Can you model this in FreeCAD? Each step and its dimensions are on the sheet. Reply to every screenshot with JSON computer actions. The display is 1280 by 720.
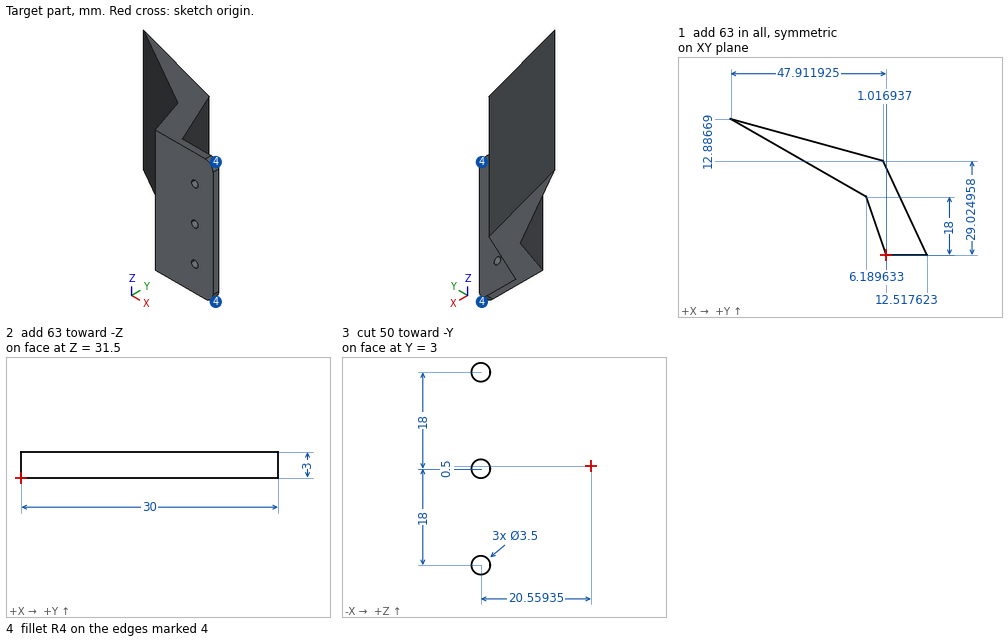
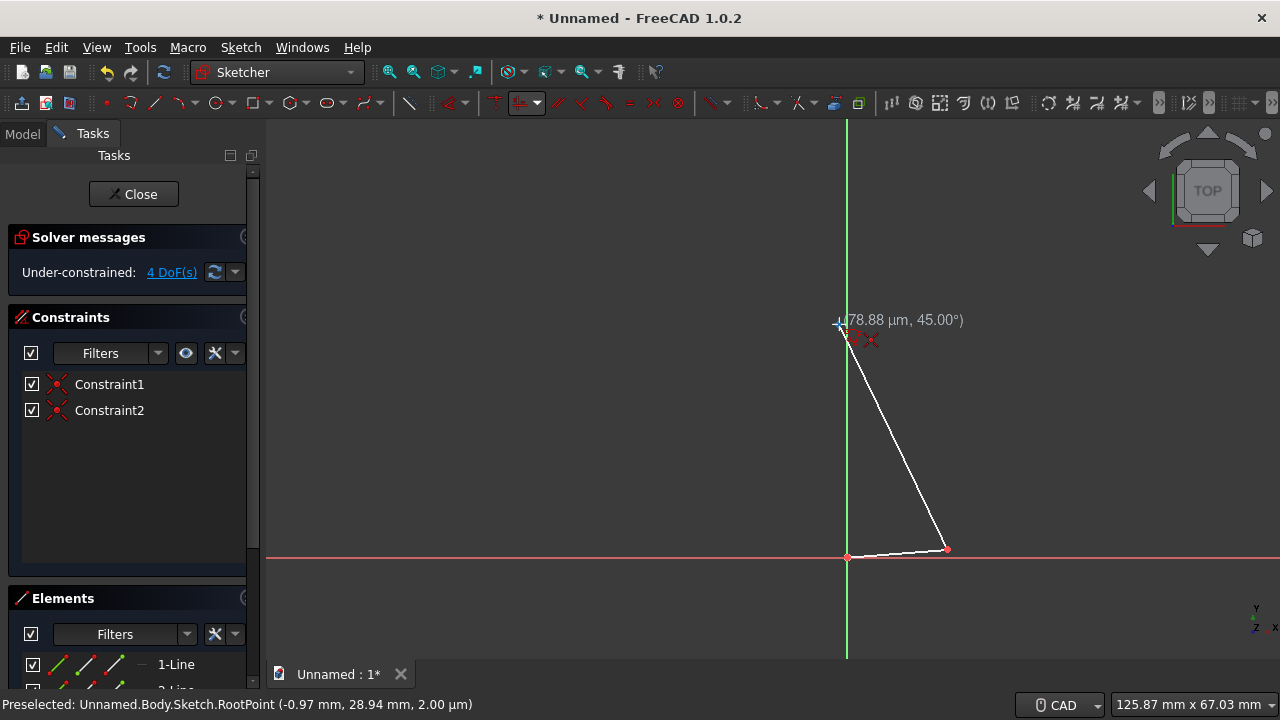
{"action": "left_click", "coordinate": [461, 220]}
{"action": "left_click", "coordinate": [797, 413]}
{"action": "left_click", "coordinate": [847, 558]}
{"action": "key", "text": "Escape"}
{"action": "key", "text": "Escape"}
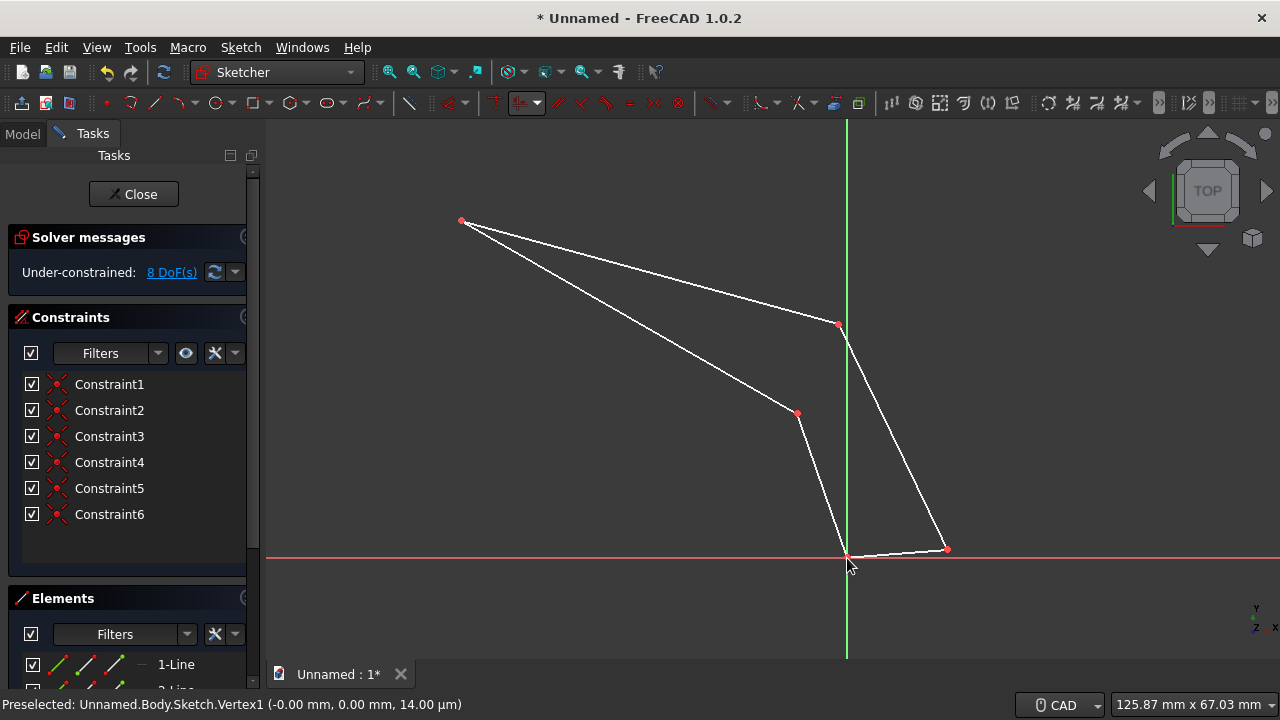
{"action": "left_click", "coordinate": [877, 555]}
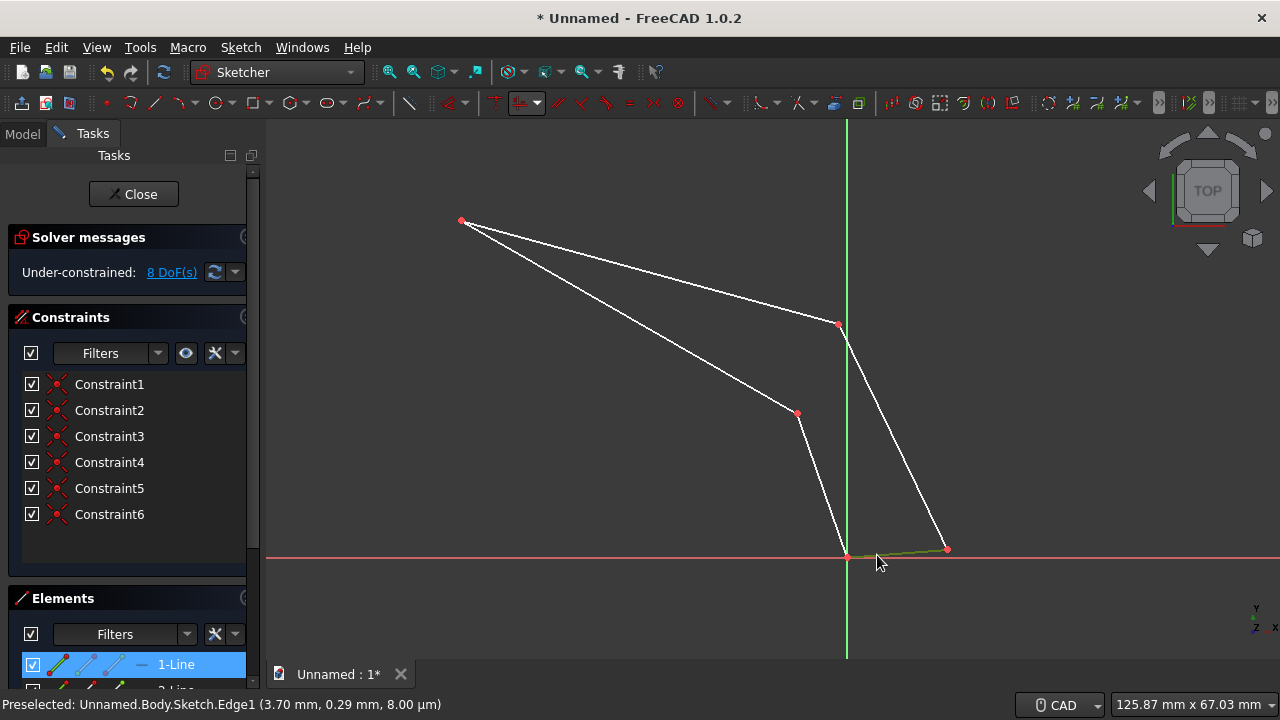
{"action": "key", "text": "h"}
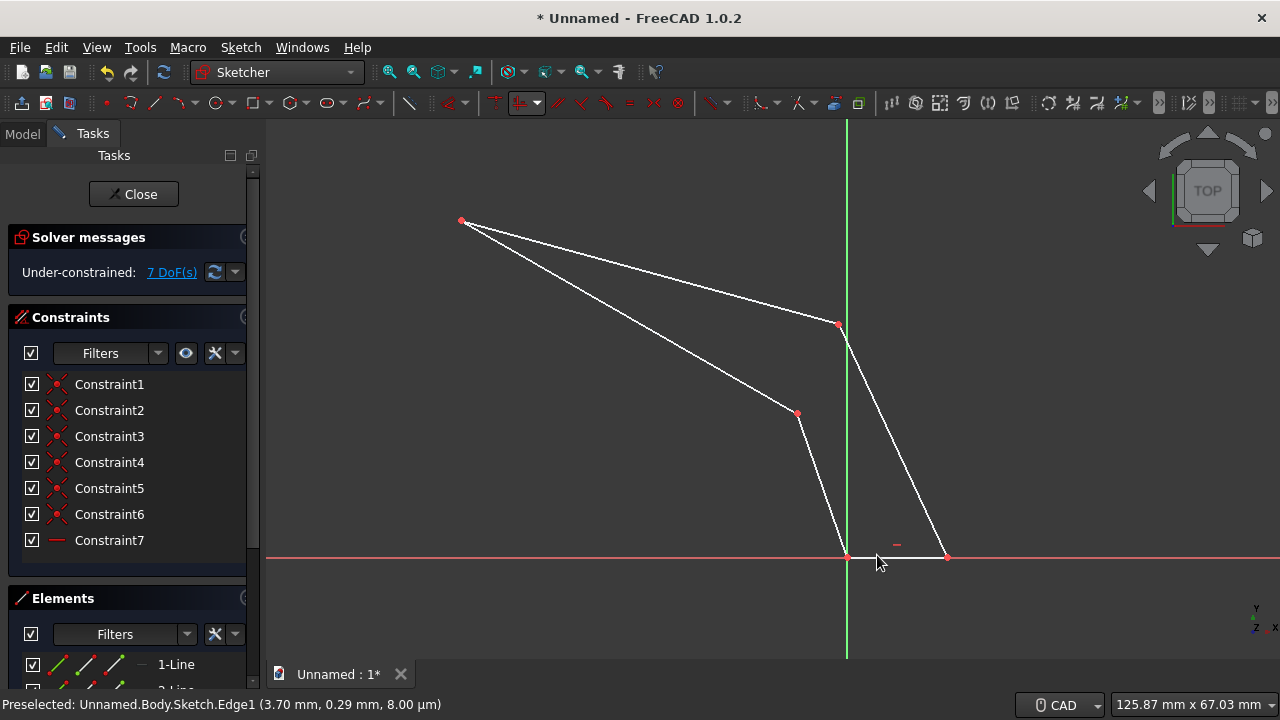
{"action": "key", "text": "d"}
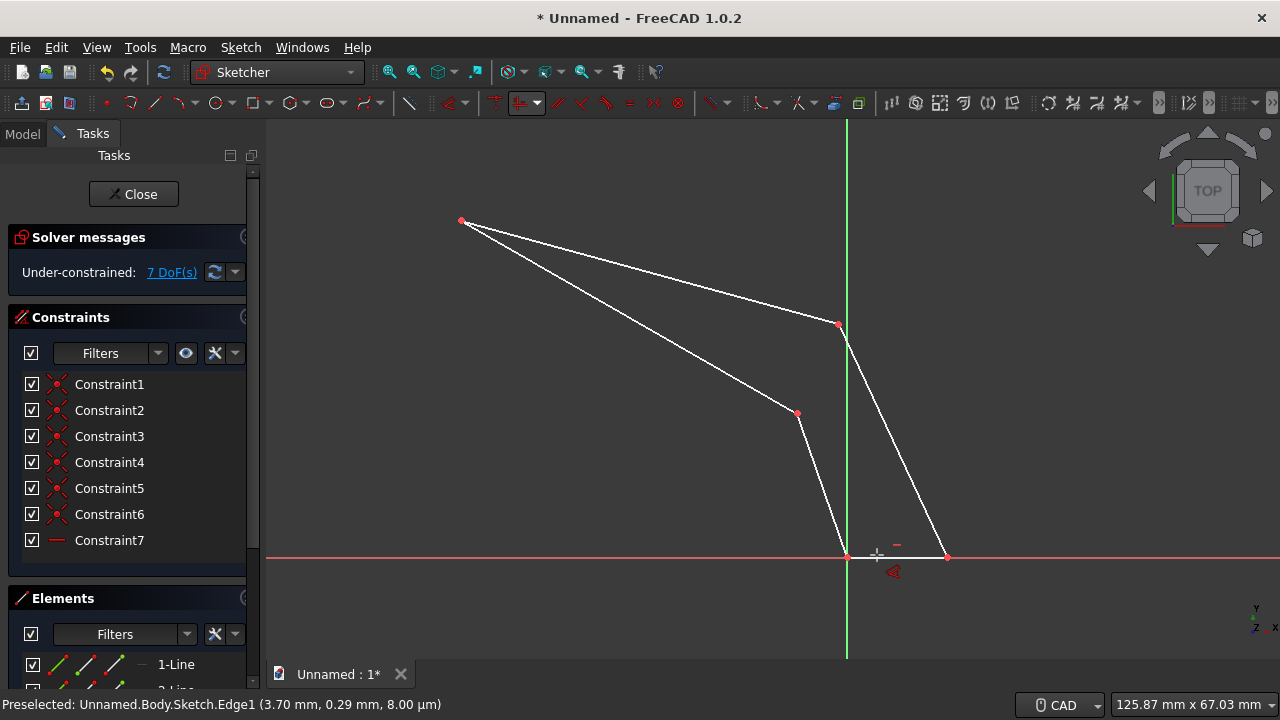
{"action": "left_click", "coordinate": [797, 414]}
{"action": "left_click", "coordinate": [881, 486]}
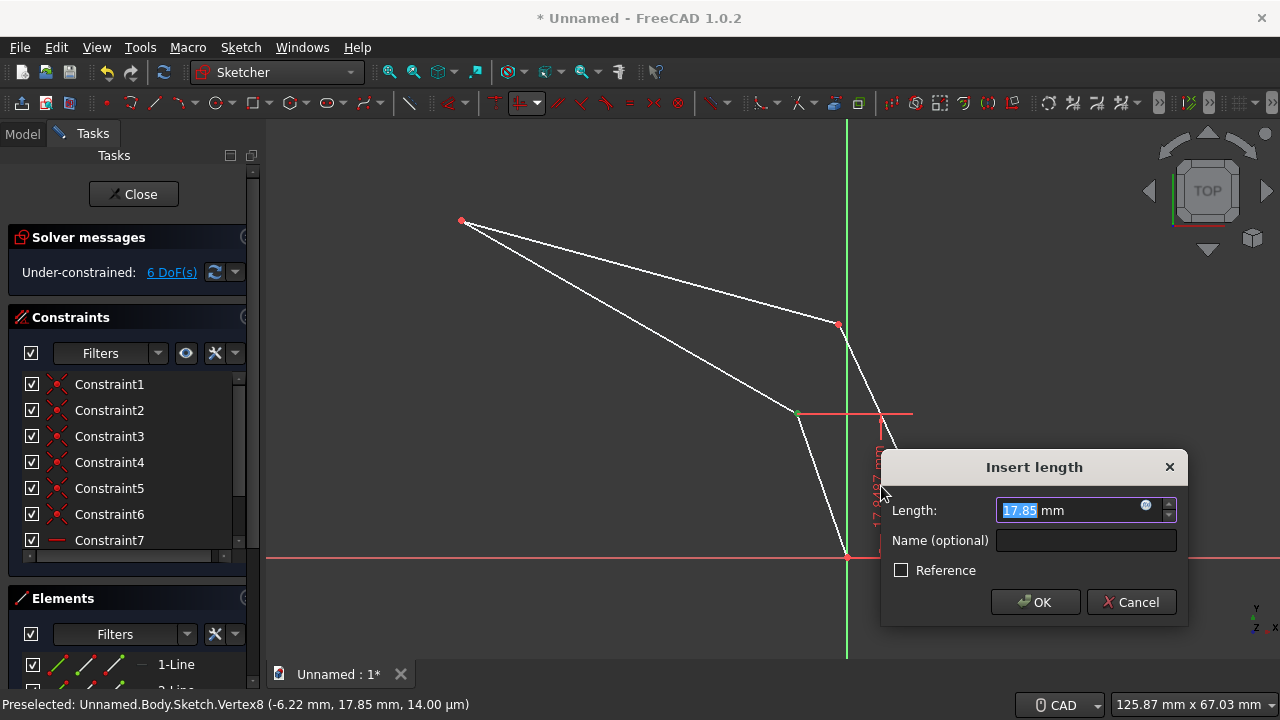
{"action": "type", "text": "18"}
{"action": "key", "text": "Return"}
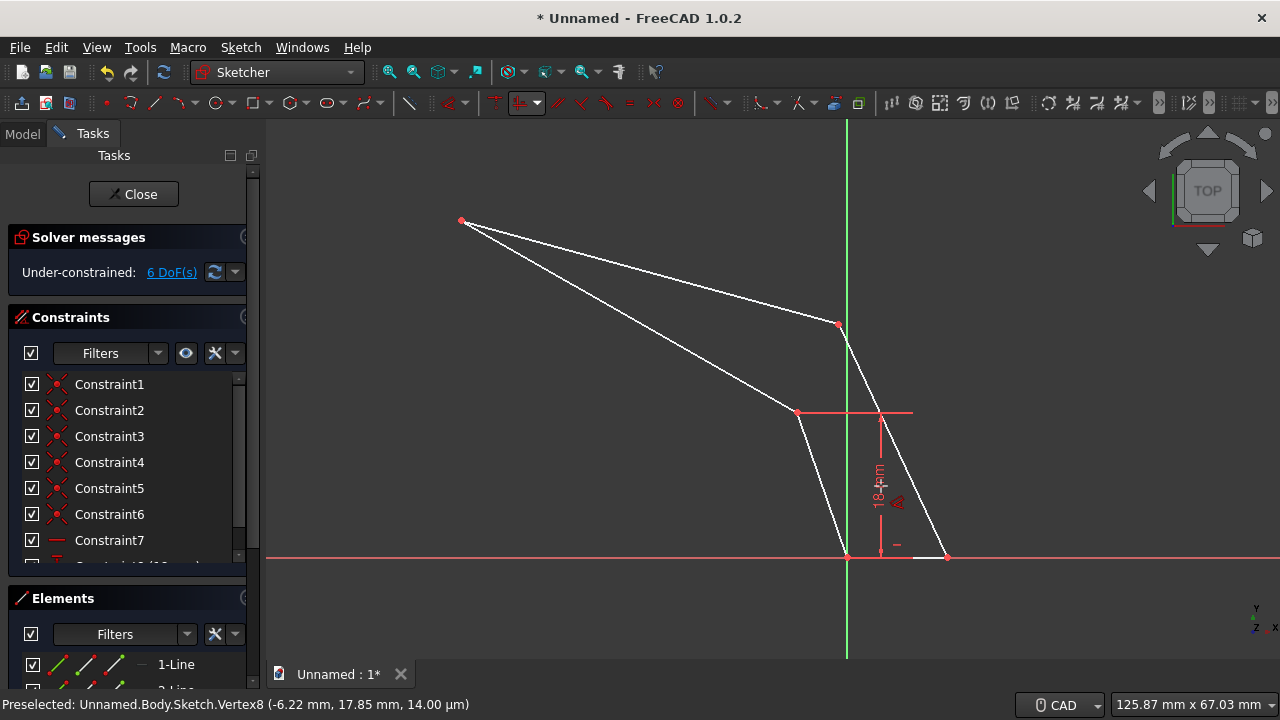
{"action": "left_click", "coordinate": [877, 558]}
{"action": "left_click", "coordinate": [897, 592]}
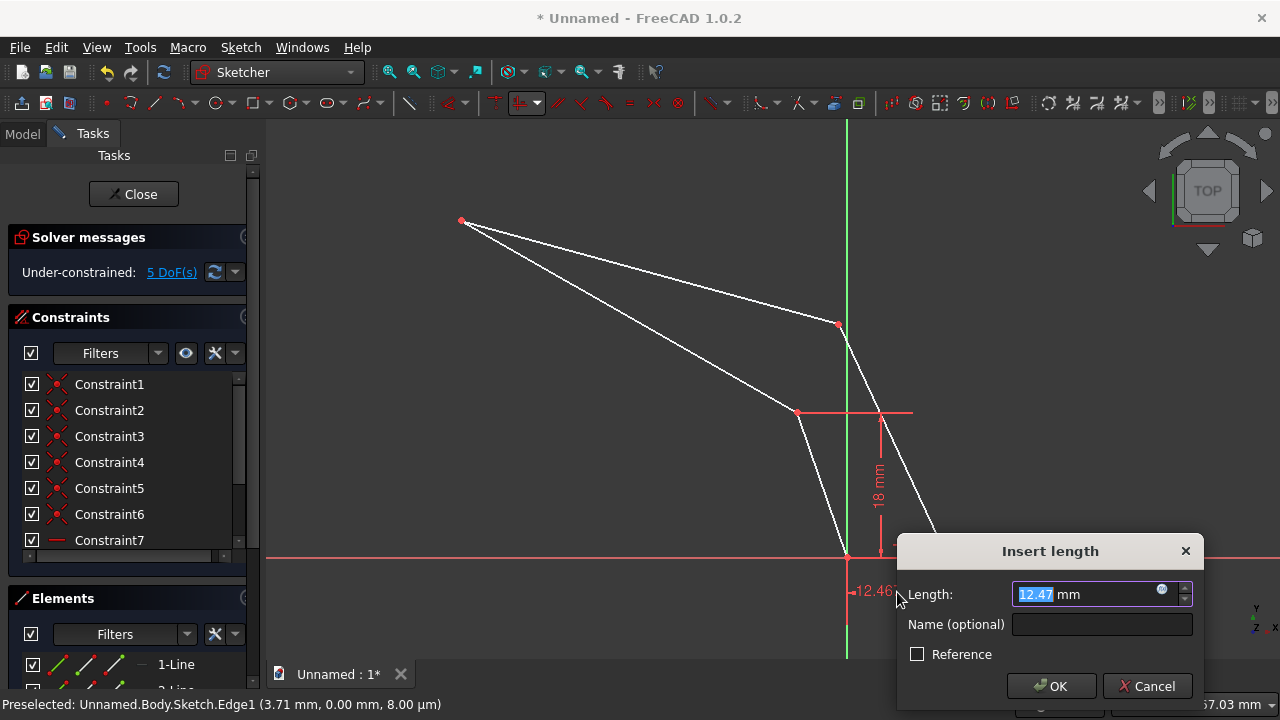
{"action": "type", "text": "12.517623"}
{"action": "key", "text": "Return"}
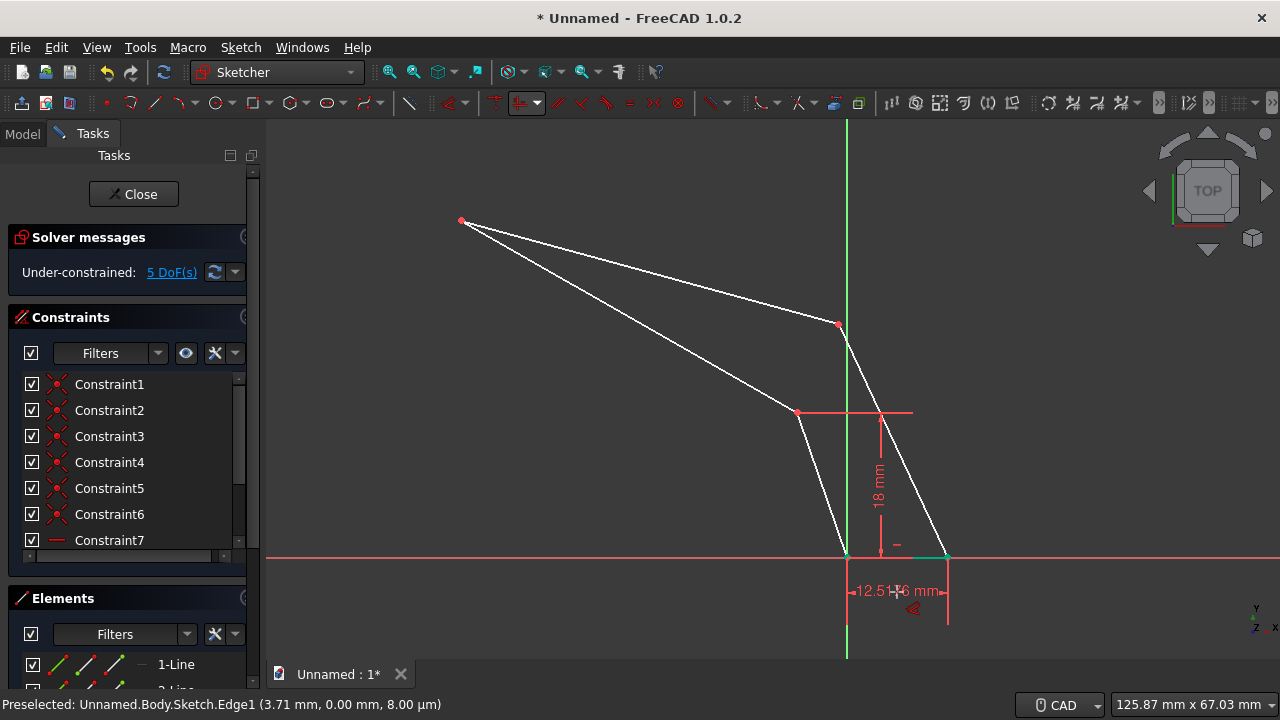
{"action": "scroll", "coordinate": [839, 324], "scroll_direction": "up", "scroll_amount": 8}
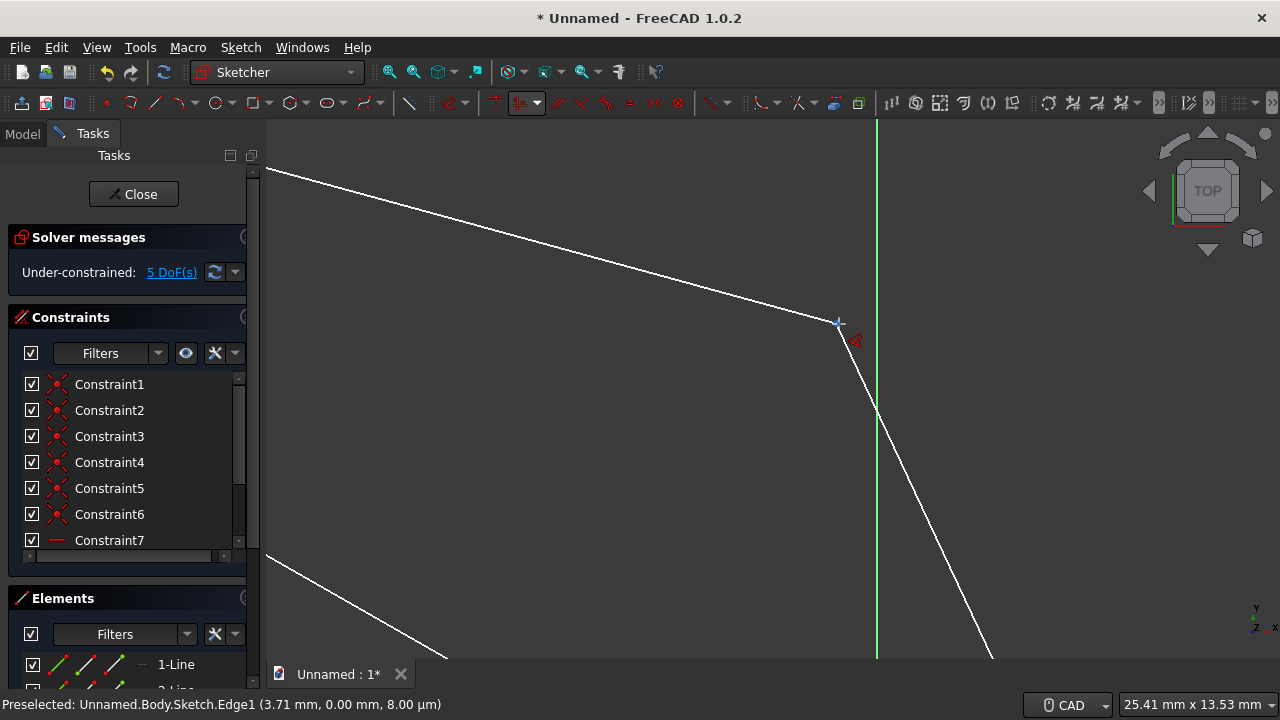
{"action": "left_click", "coordinate": [836, 324]}
{"action": "left_click", "coordinate": [857, 290]}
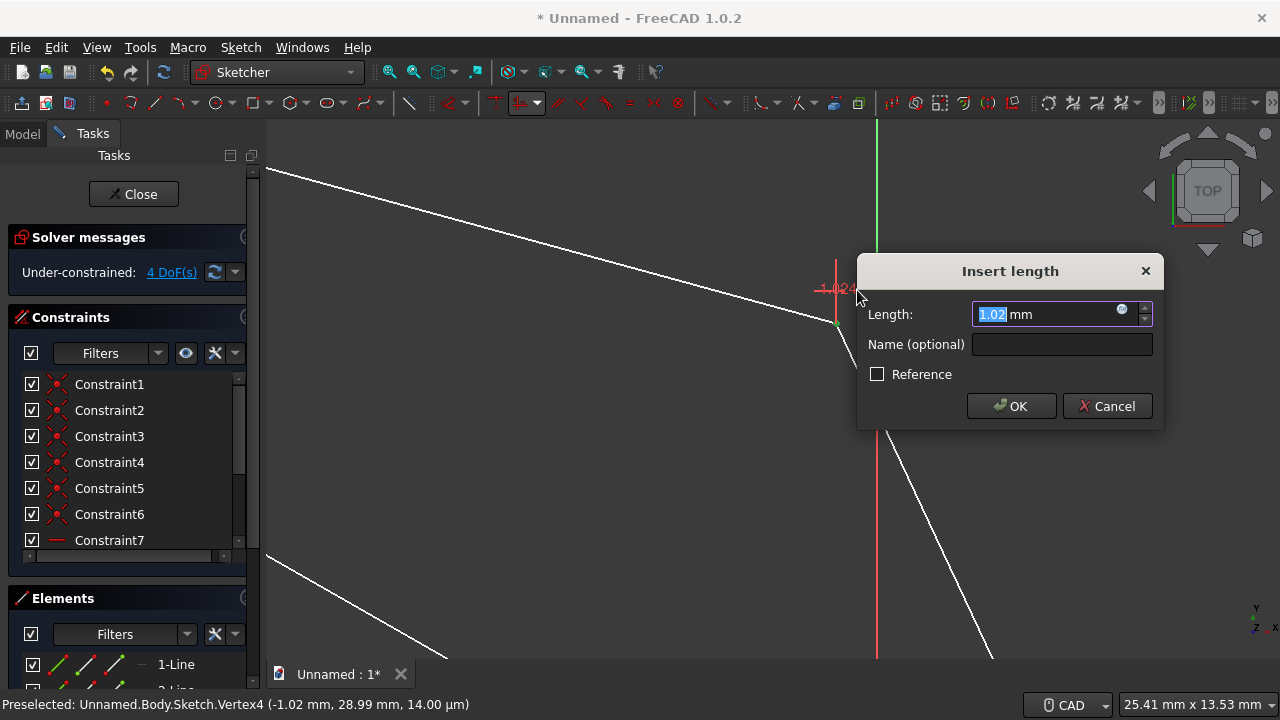
{"action": "type", "text": "1.016937"}
{"action": "key", "text": "Return"}